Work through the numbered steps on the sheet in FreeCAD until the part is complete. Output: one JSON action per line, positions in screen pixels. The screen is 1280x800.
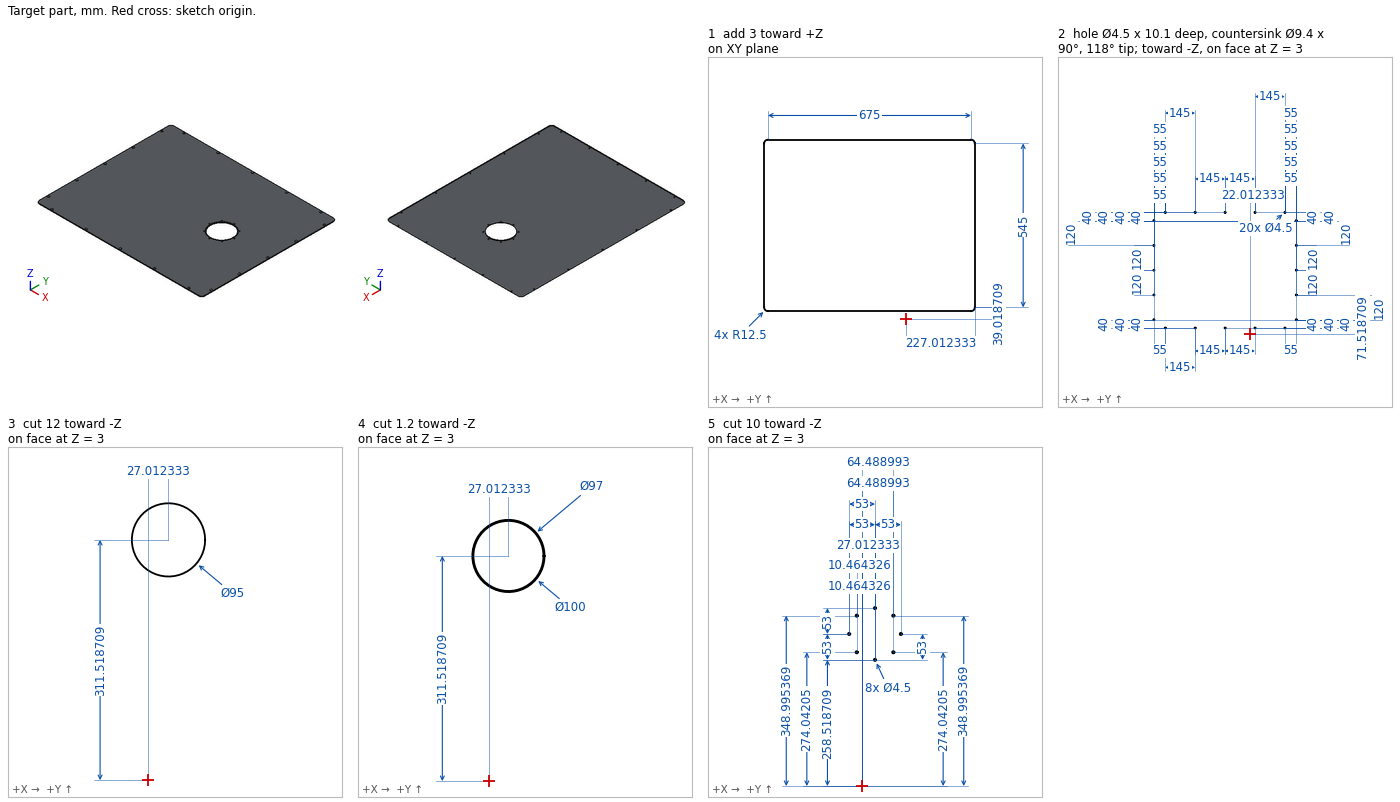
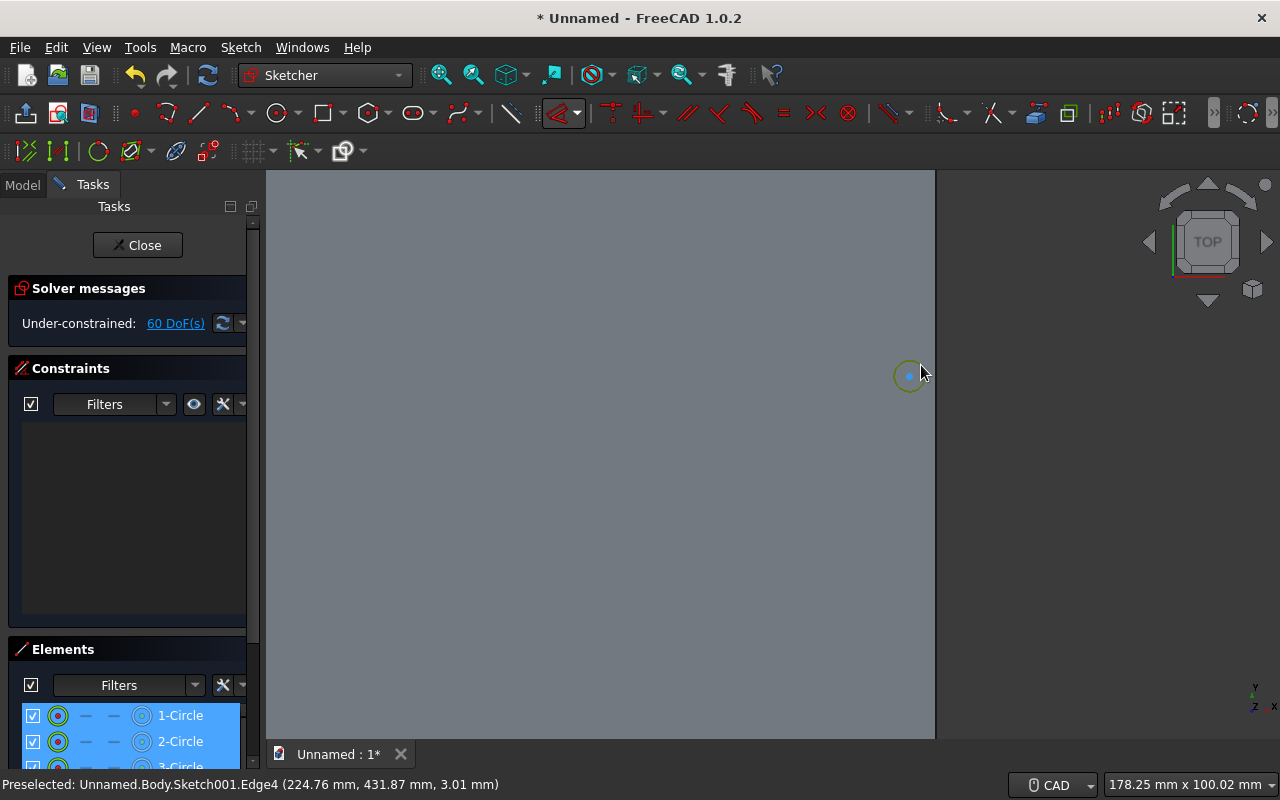
{"action": "scroll", "coordinate": [924, 370], "scroll_direction": "down", "scroll_amount": 11}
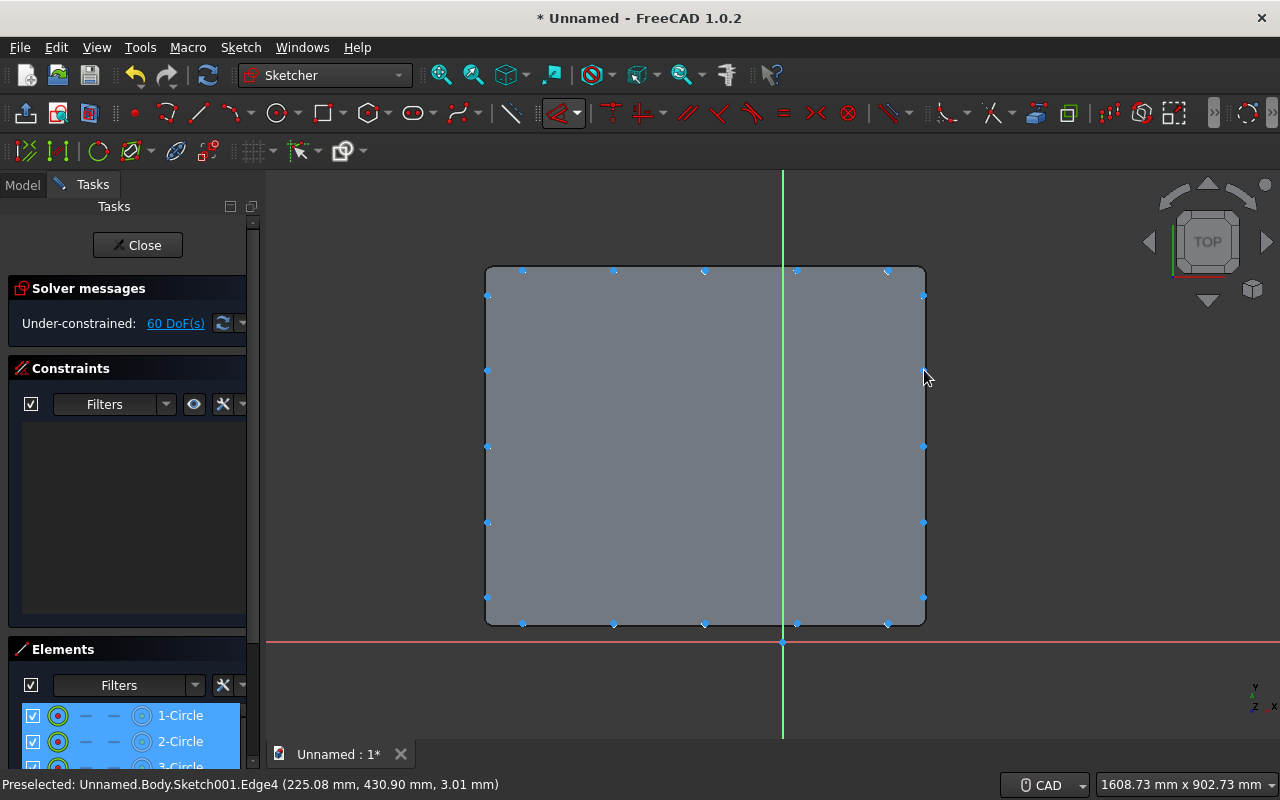
{"action": "scroll", "coordinate": [925, 294], "scroll_direction": "up", "scroll_amount": 10}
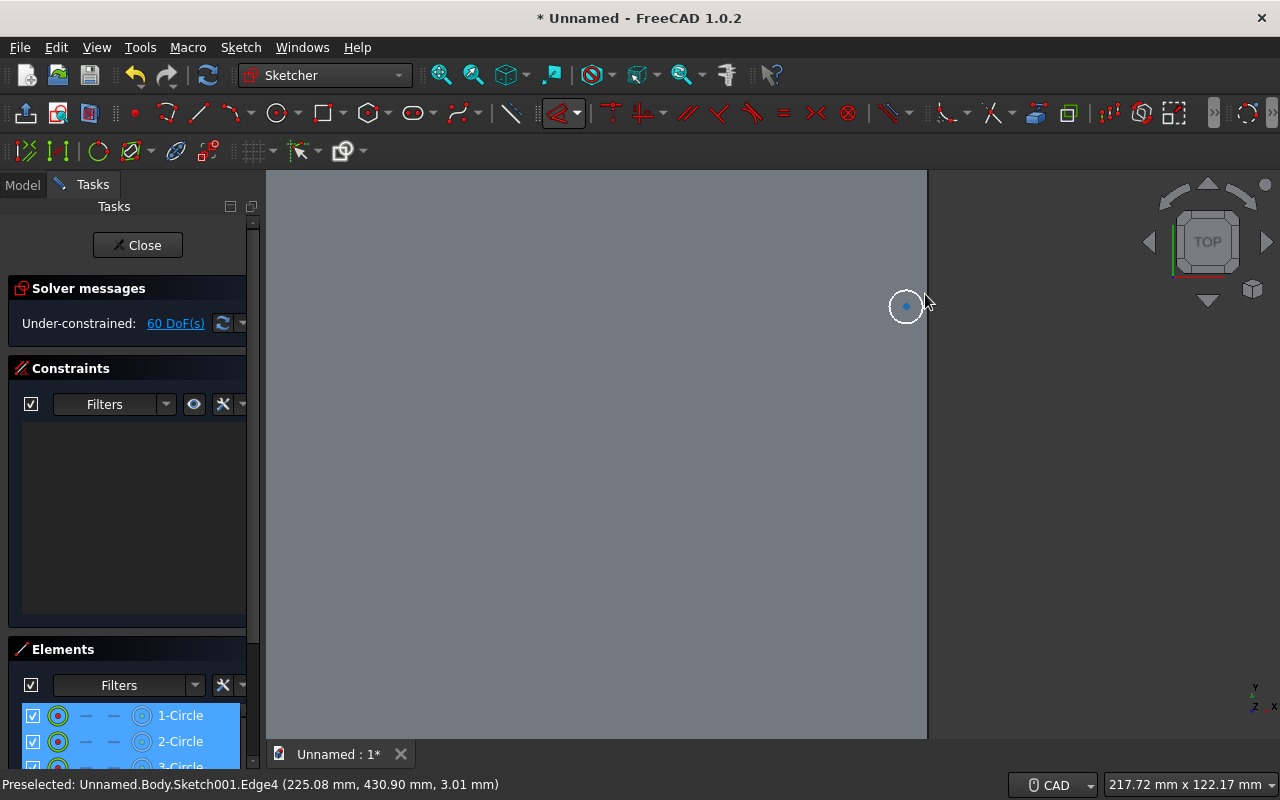
{"action": "left_click", "coordinate": [918, 295]}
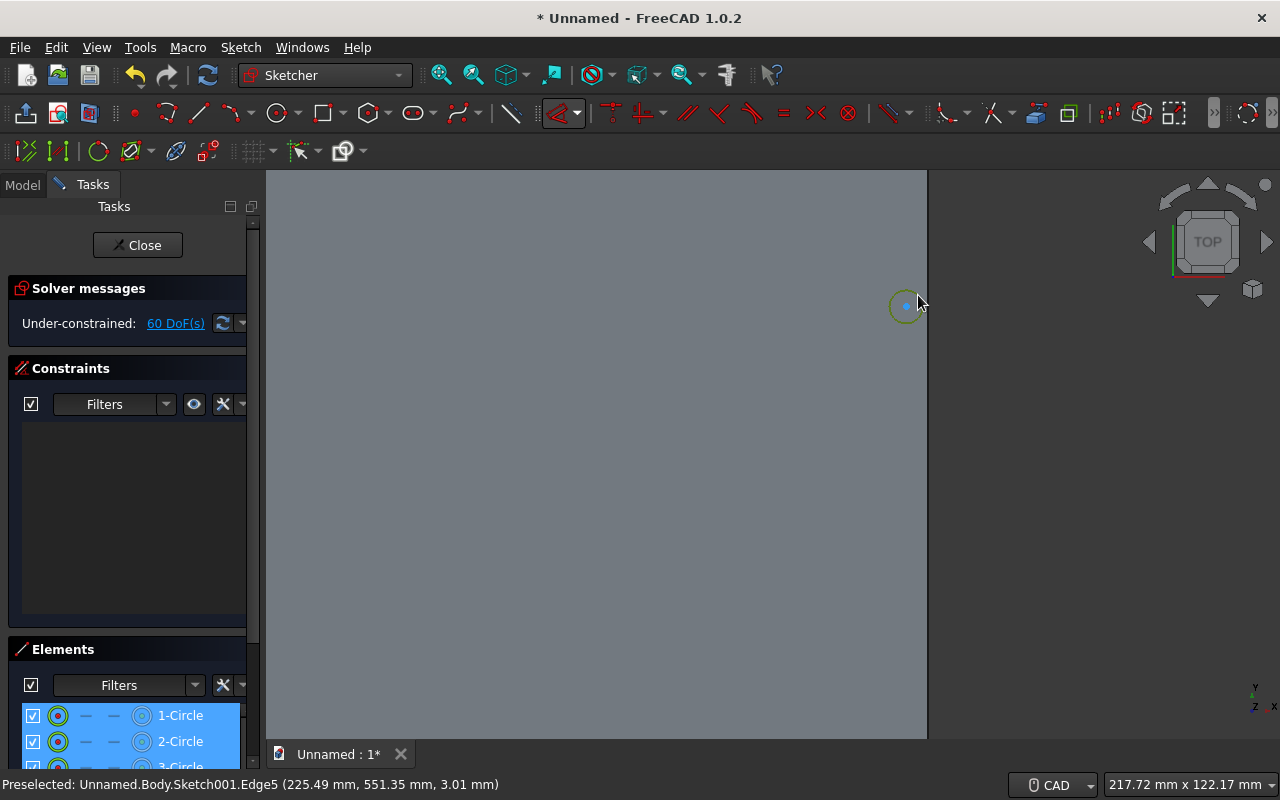
{"action": "scroll", "coordinate": [925, 293], "scroll_direction": "down", "scroll_amount": 10}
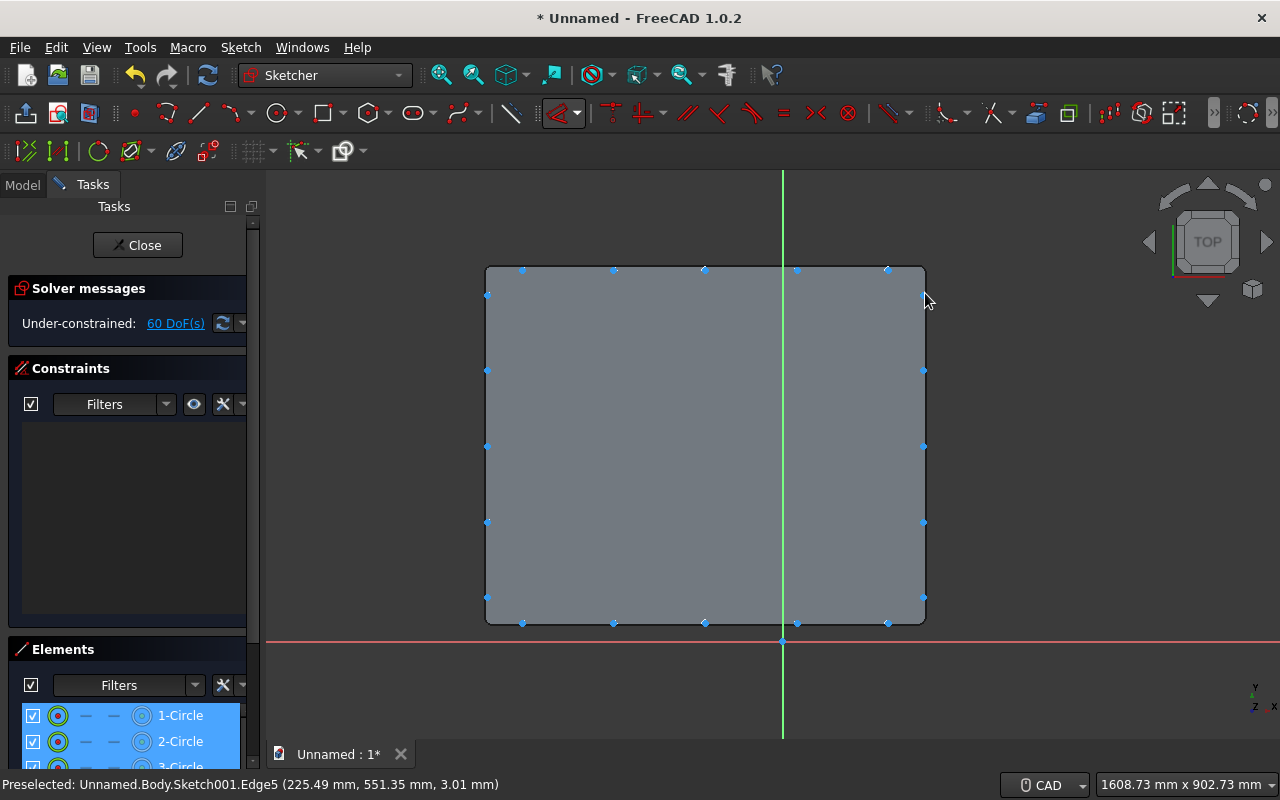
{"action": "scroll", "coordinate": [890, 268], "scroll_direction": "up", "scroll_amount": 9}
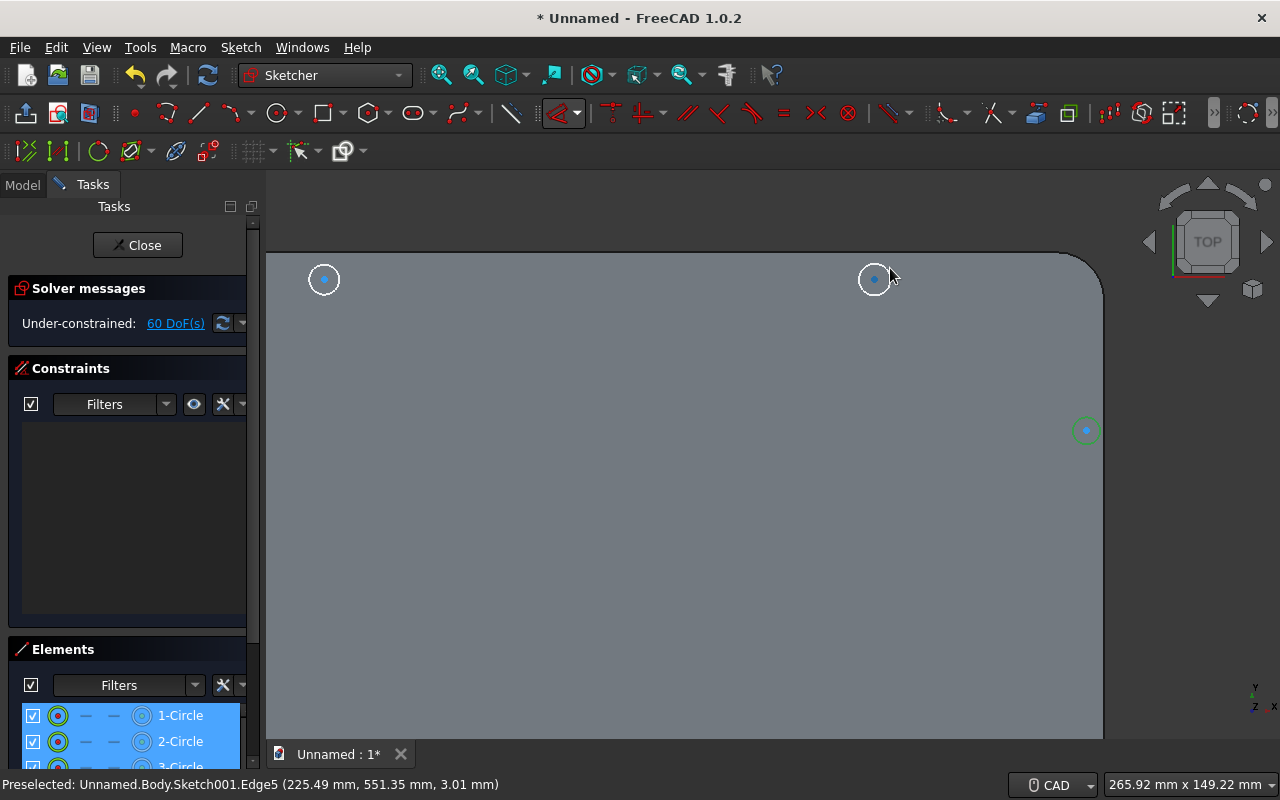
{"action": "left_click", "coordinate": [886, 268]}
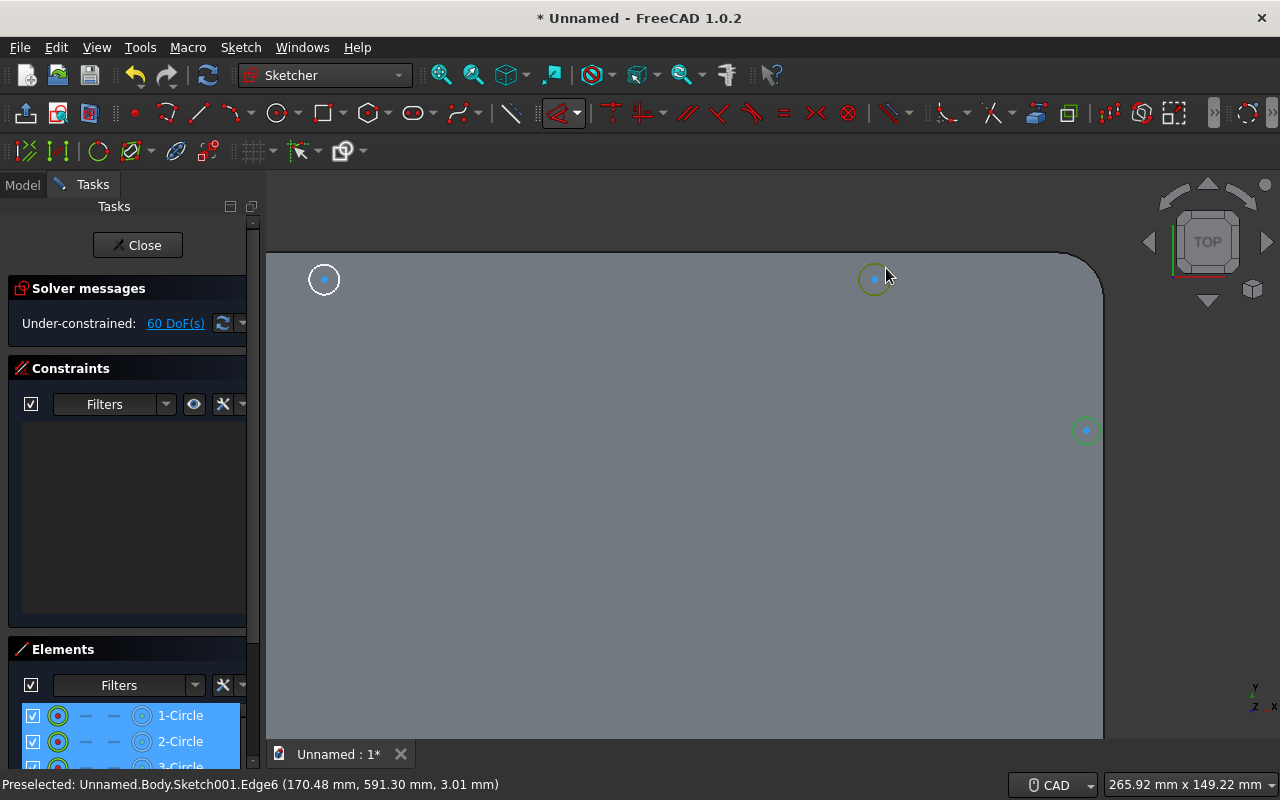
{"action": "left_click", "coordinate": [335, 269]}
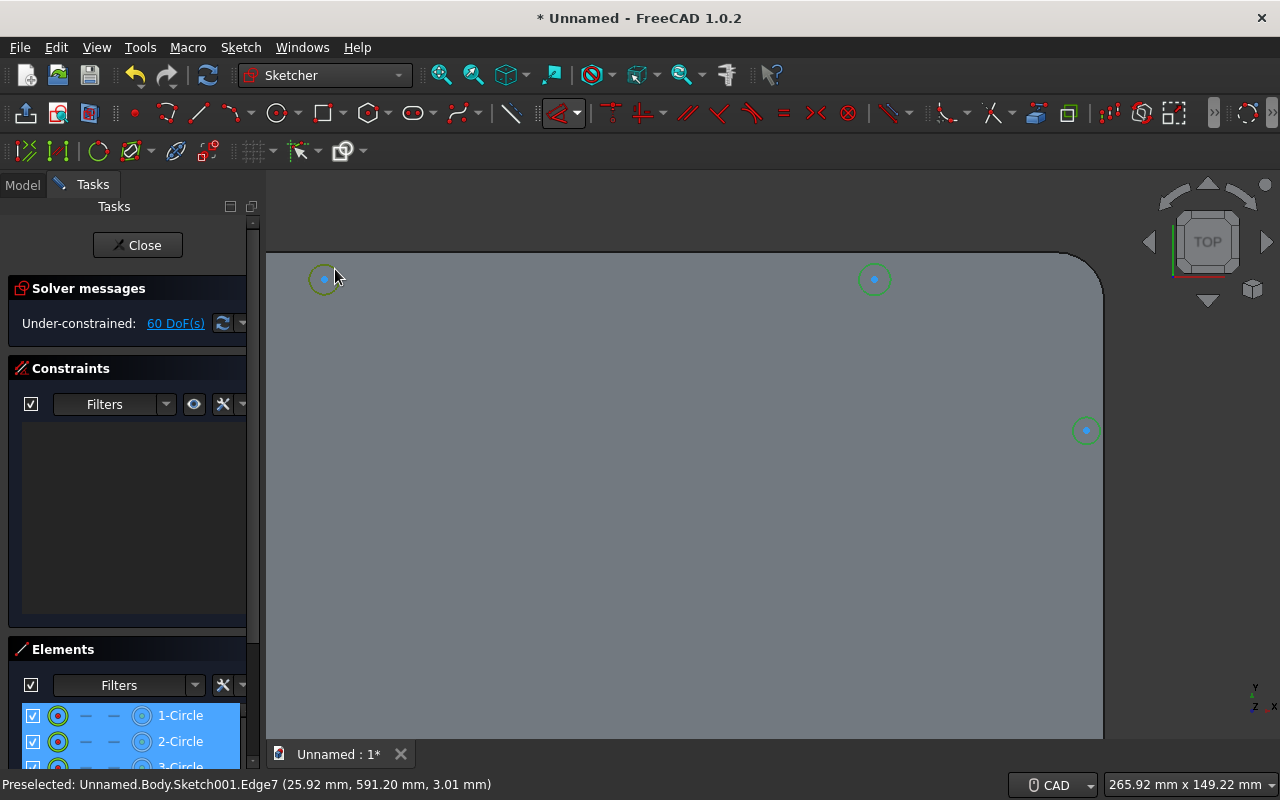
{"action": "scroll", "coordinate": [890, 268], "scroll_direction": "down", "scroll_amount": 9}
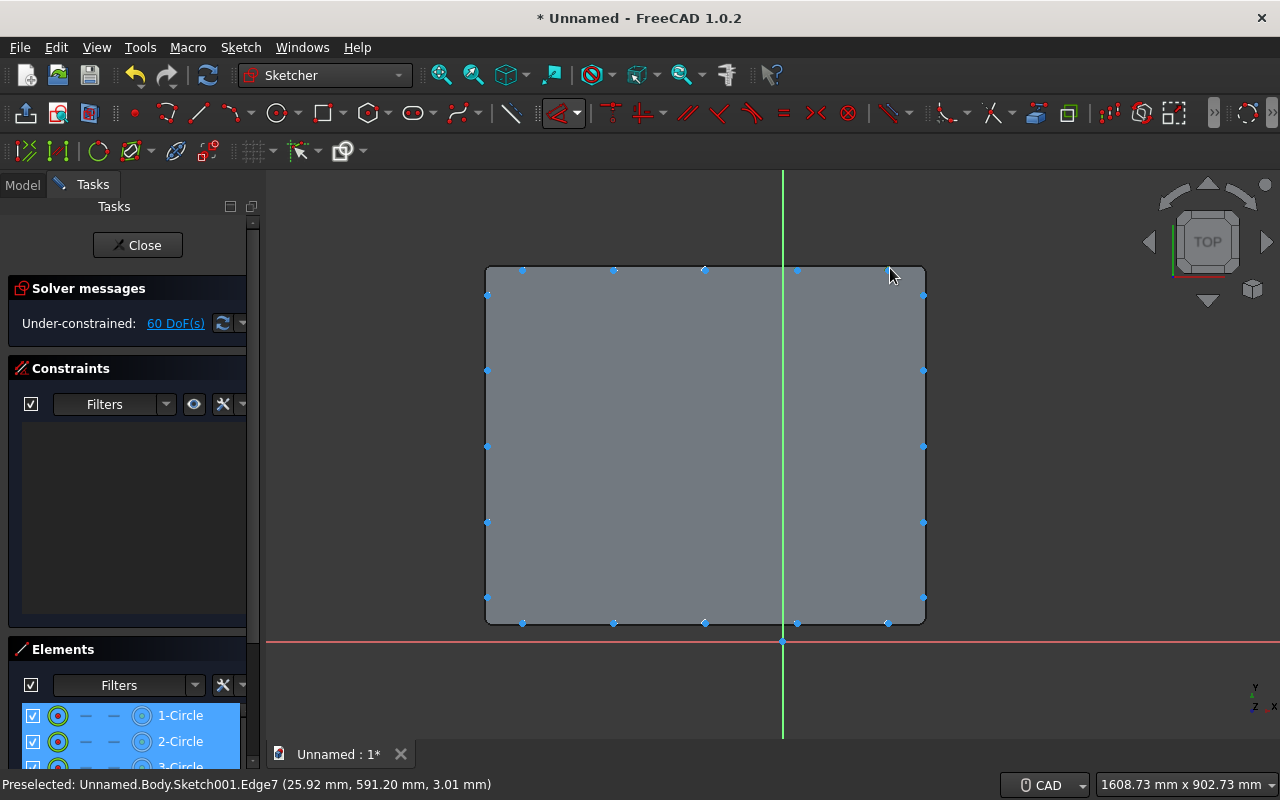
{"action": "scroll", "coordinate": [707, 268], "scroll_direction": "up", "scroll_amount": 9}